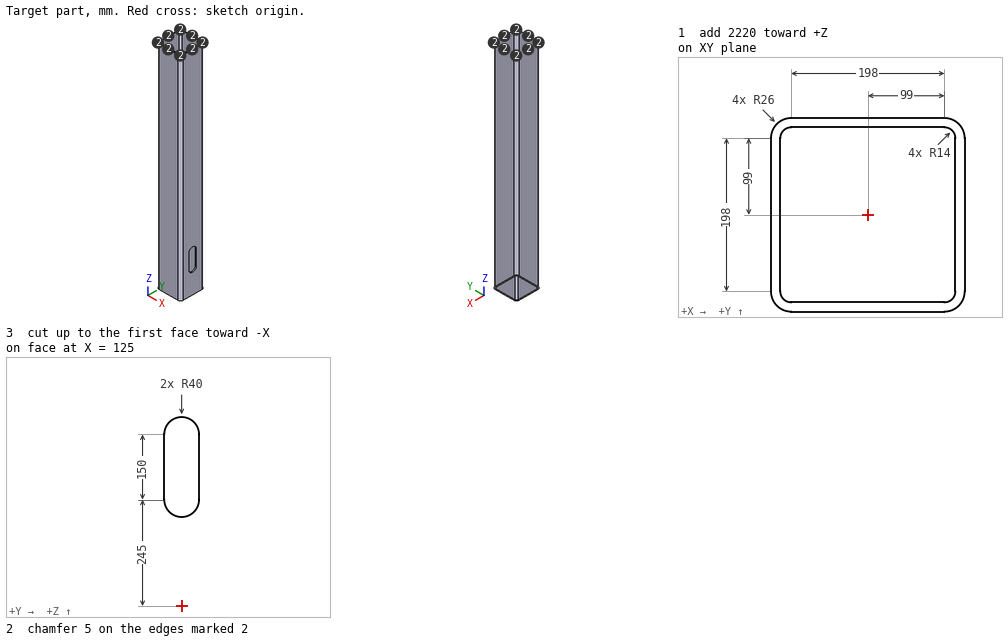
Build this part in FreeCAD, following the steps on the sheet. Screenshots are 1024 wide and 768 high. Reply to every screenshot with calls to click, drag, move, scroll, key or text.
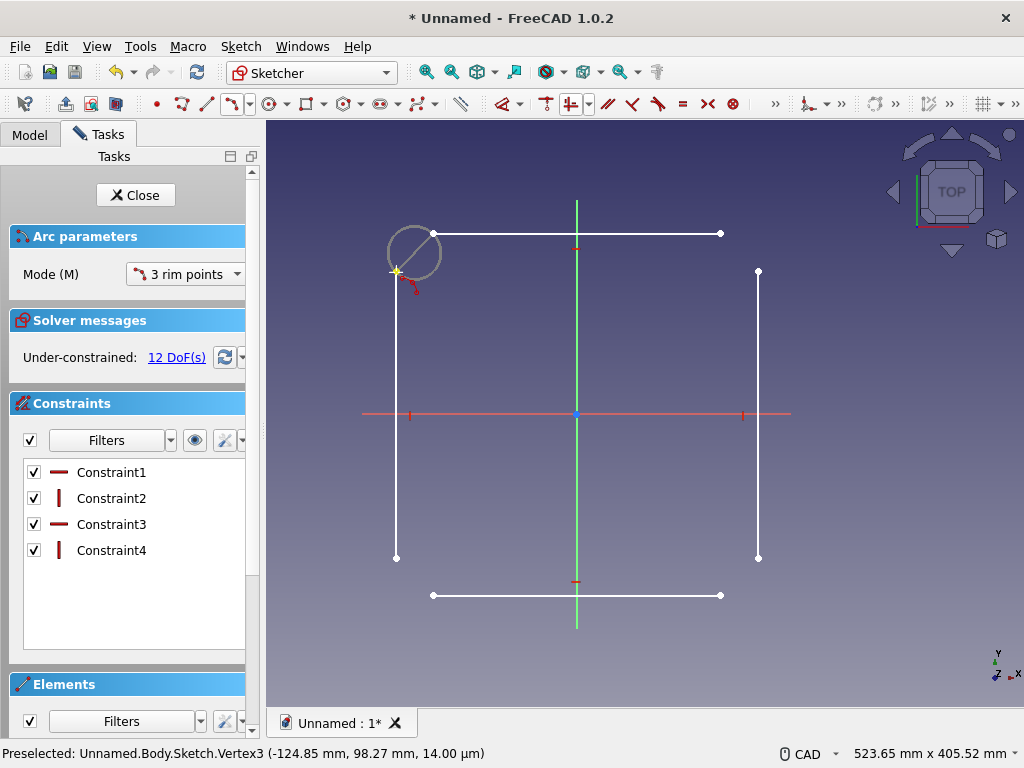
scroll(407, 244, up, 2)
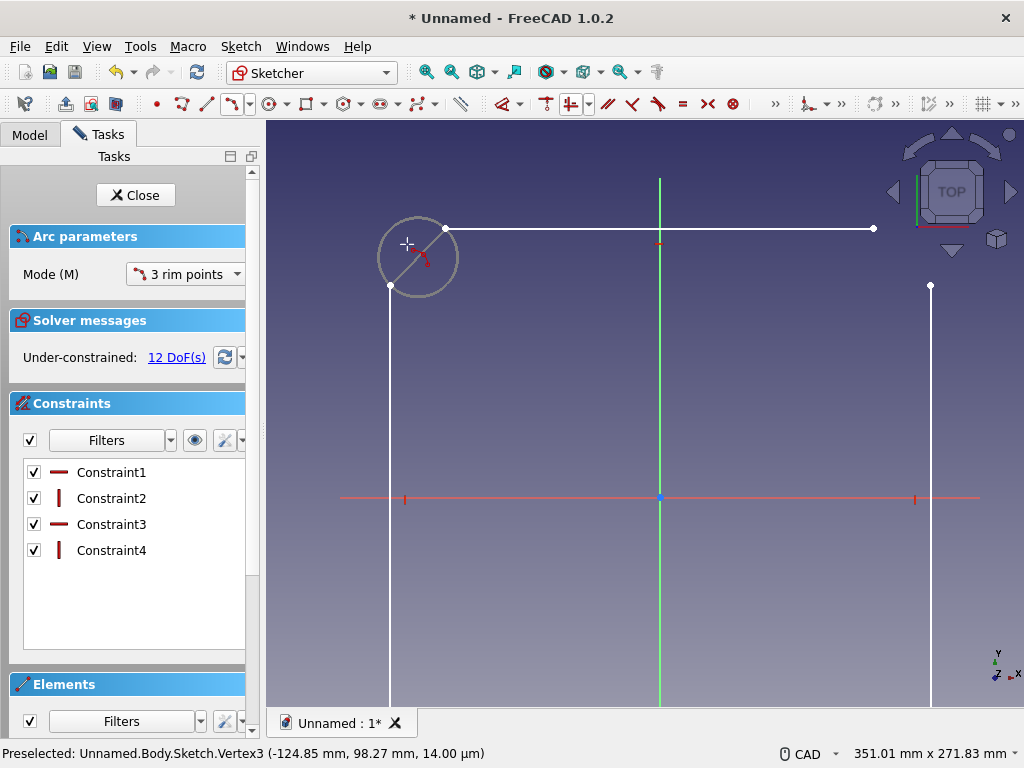
click(407, 244)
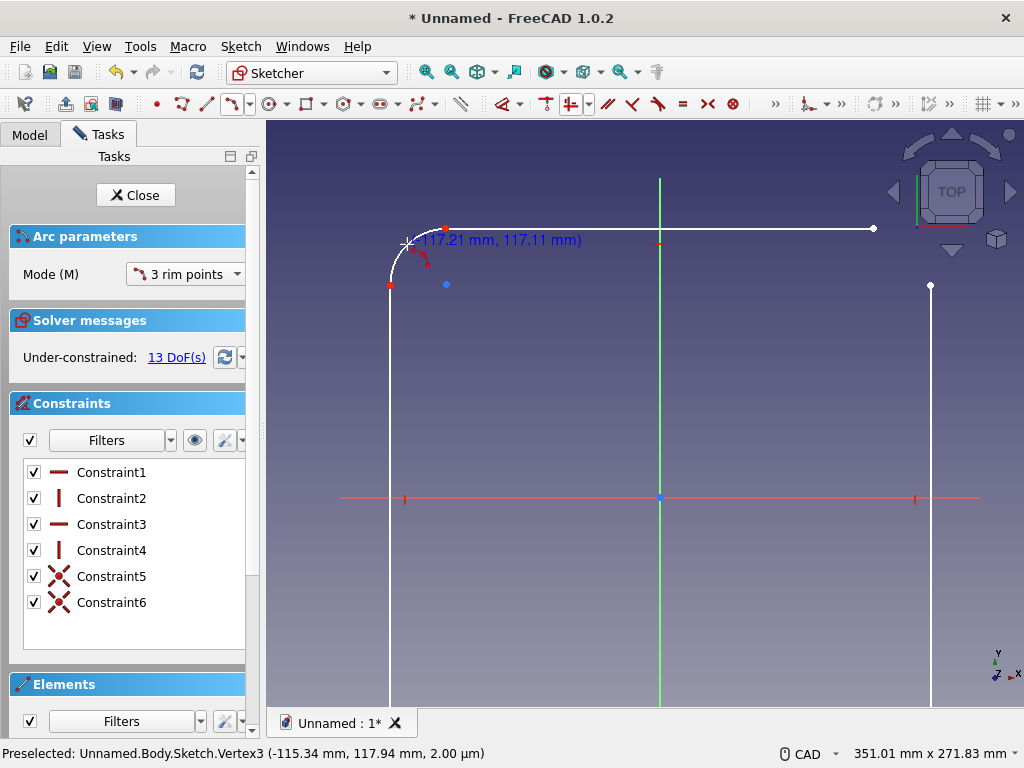
scroll(406, 242, down, 2)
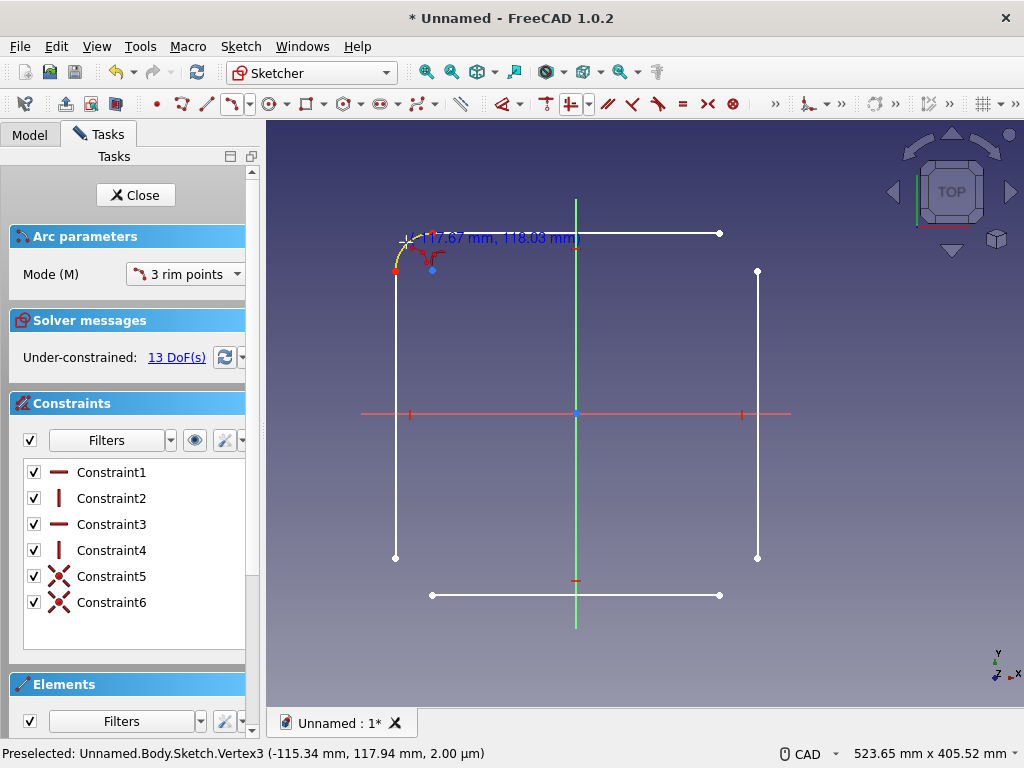
click(396, 558)
click(433, 595)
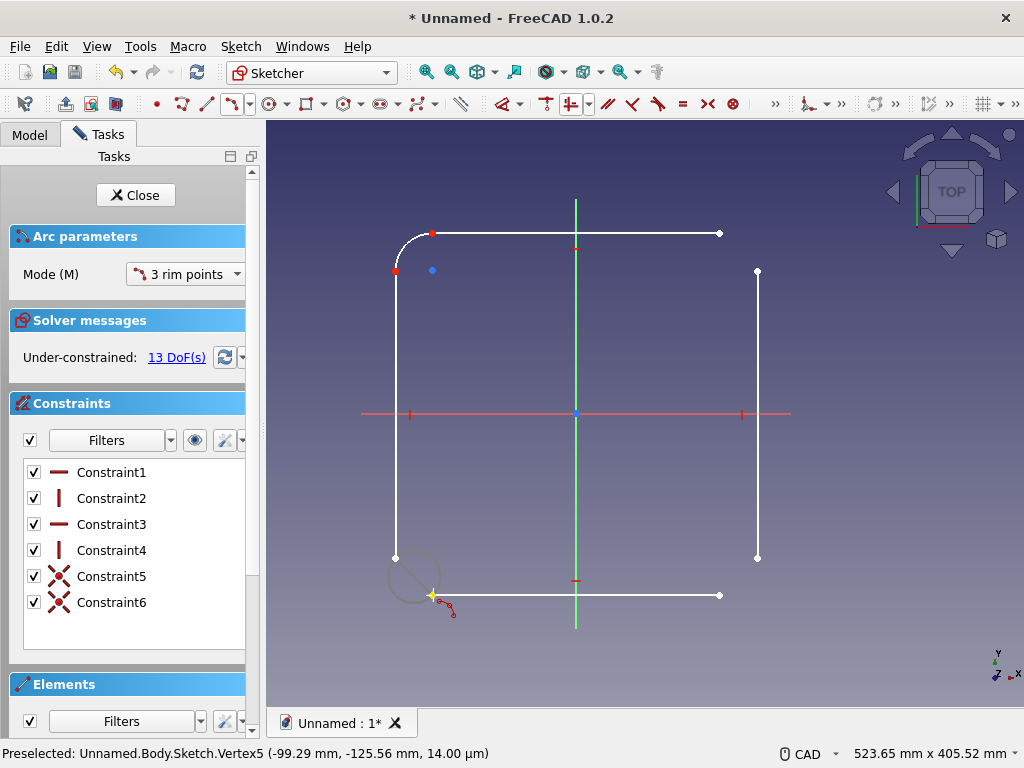
scroll(406, 584, up, 2)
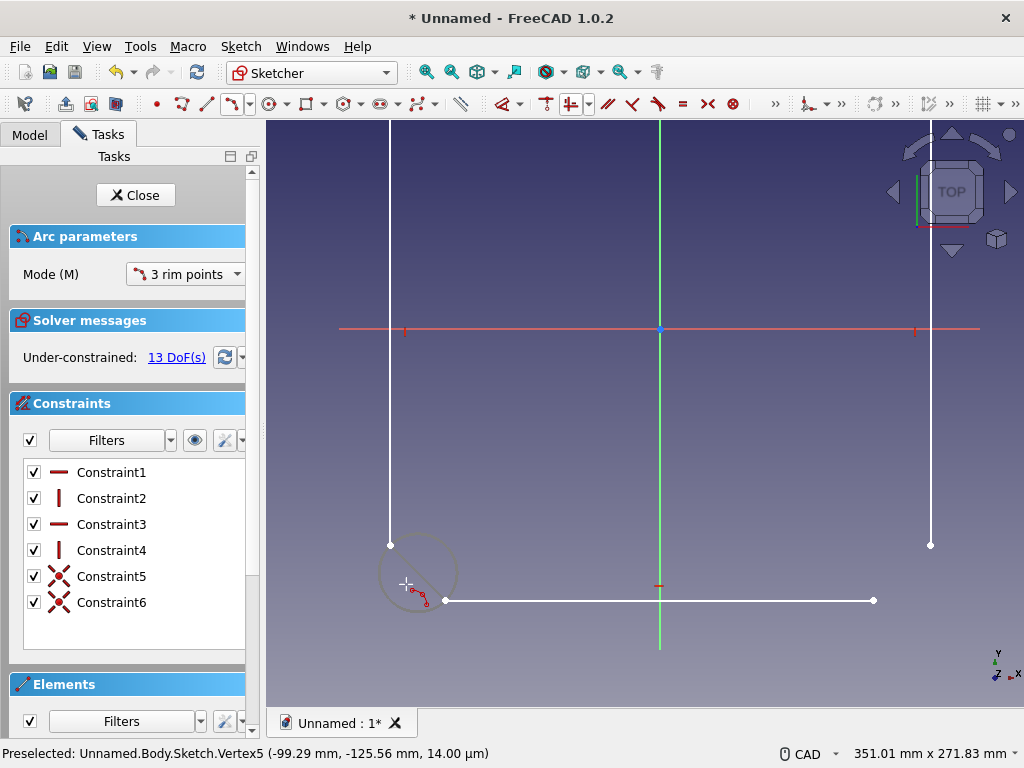
click(407, 583)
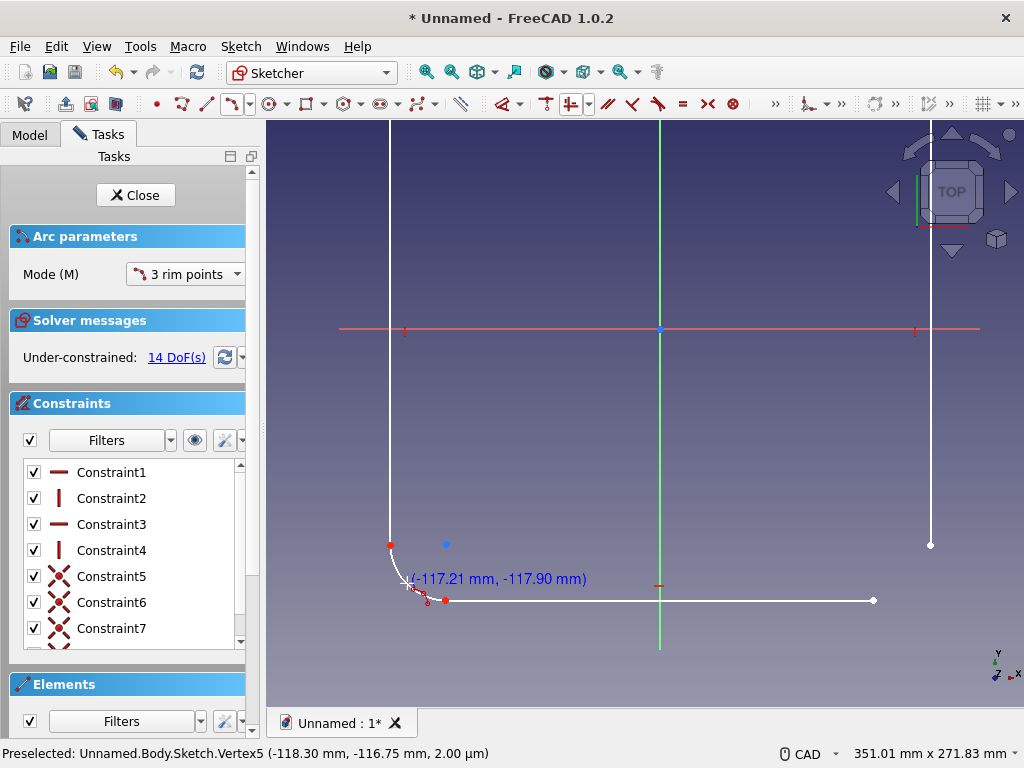
scroll(406, 585, down, 2)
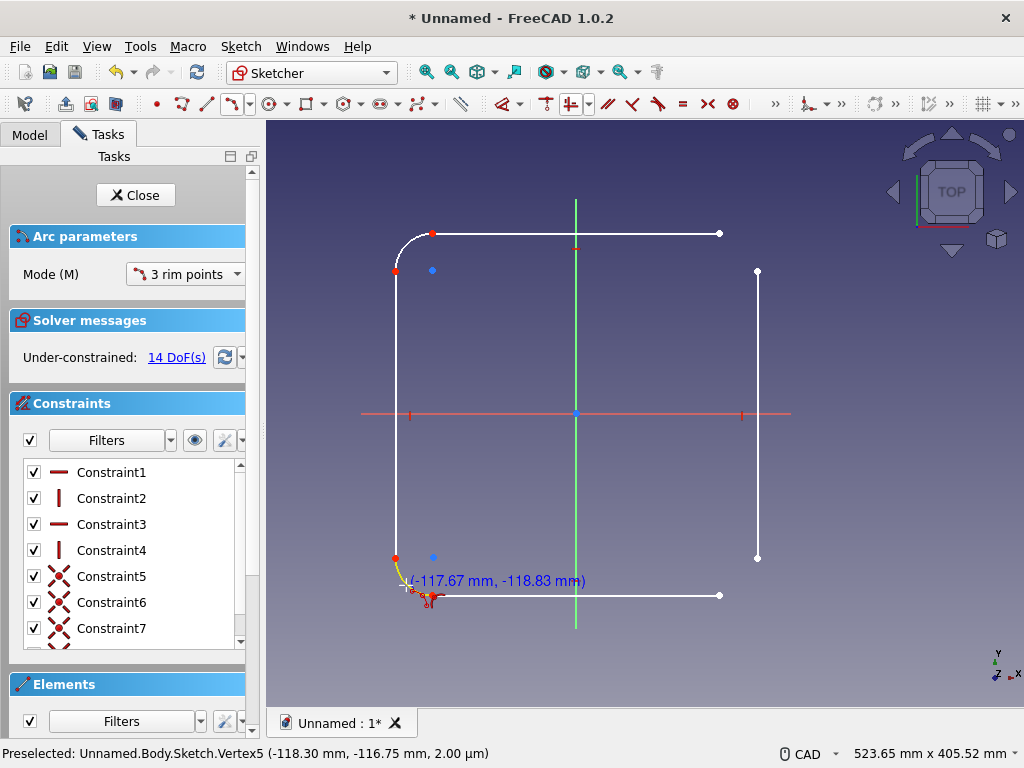
click(720, 596)
click(758, 559)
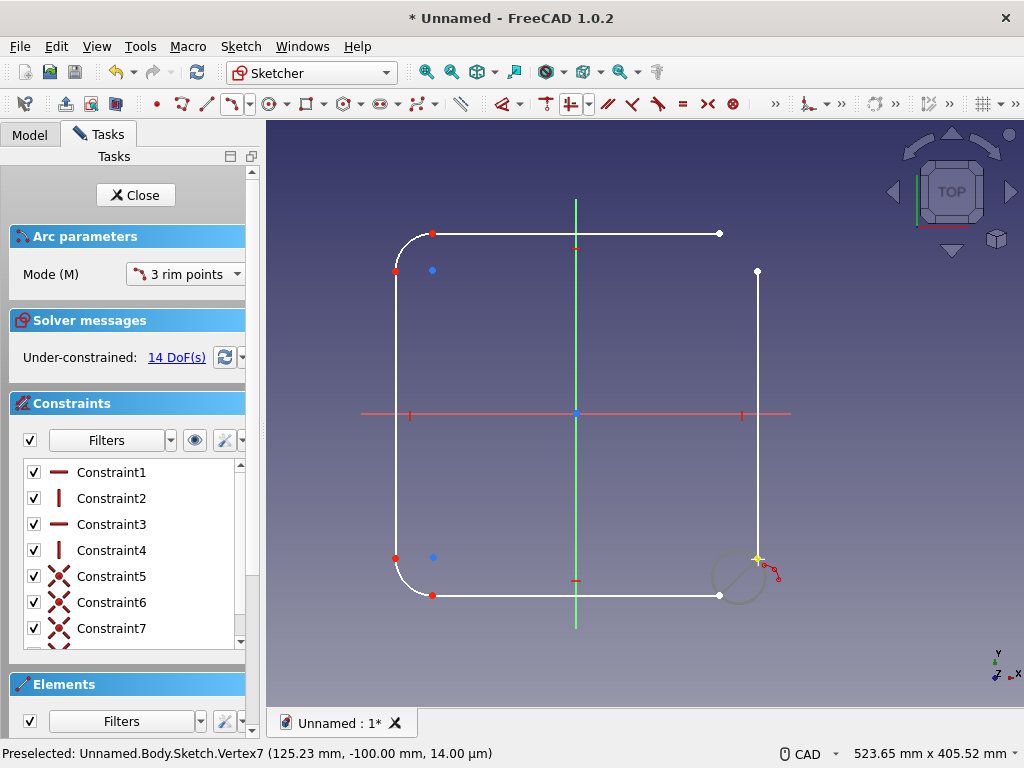
scroll(746, 584, up, 2)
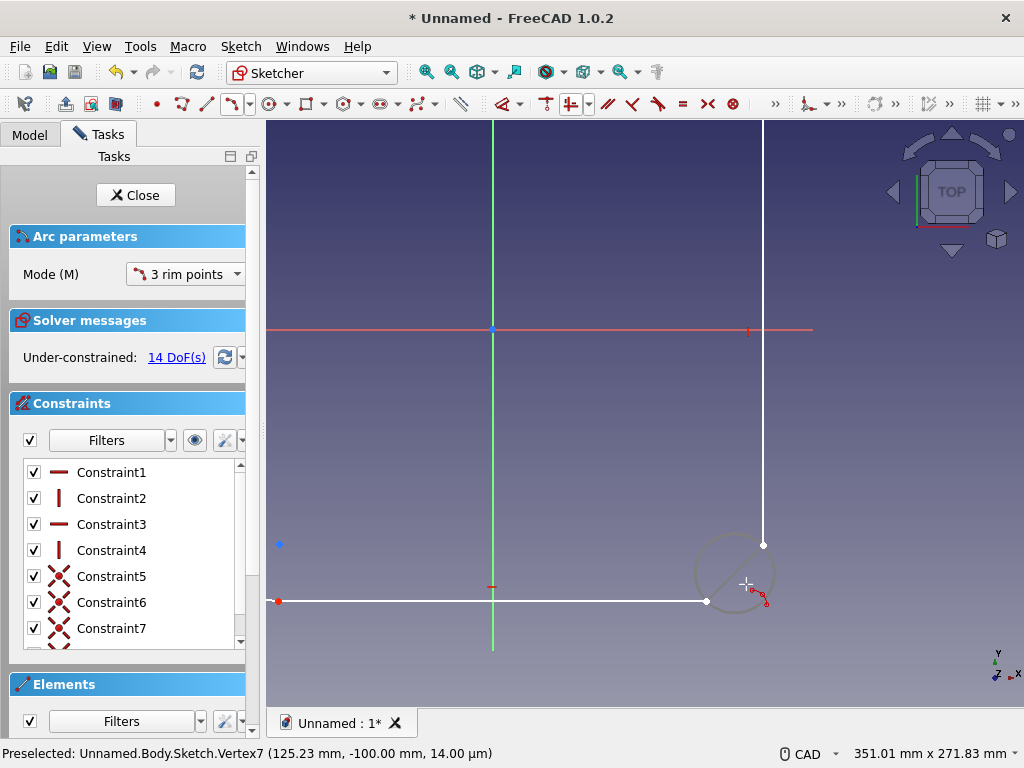
click(746, 583)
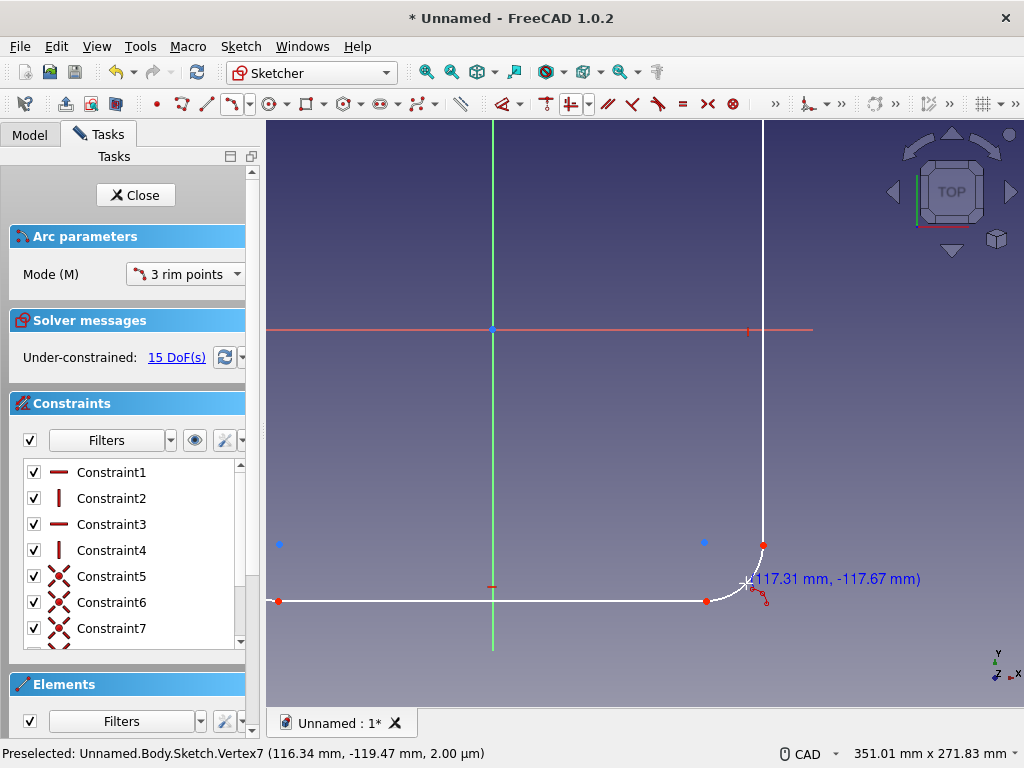
scroll(747, 584, down, 2)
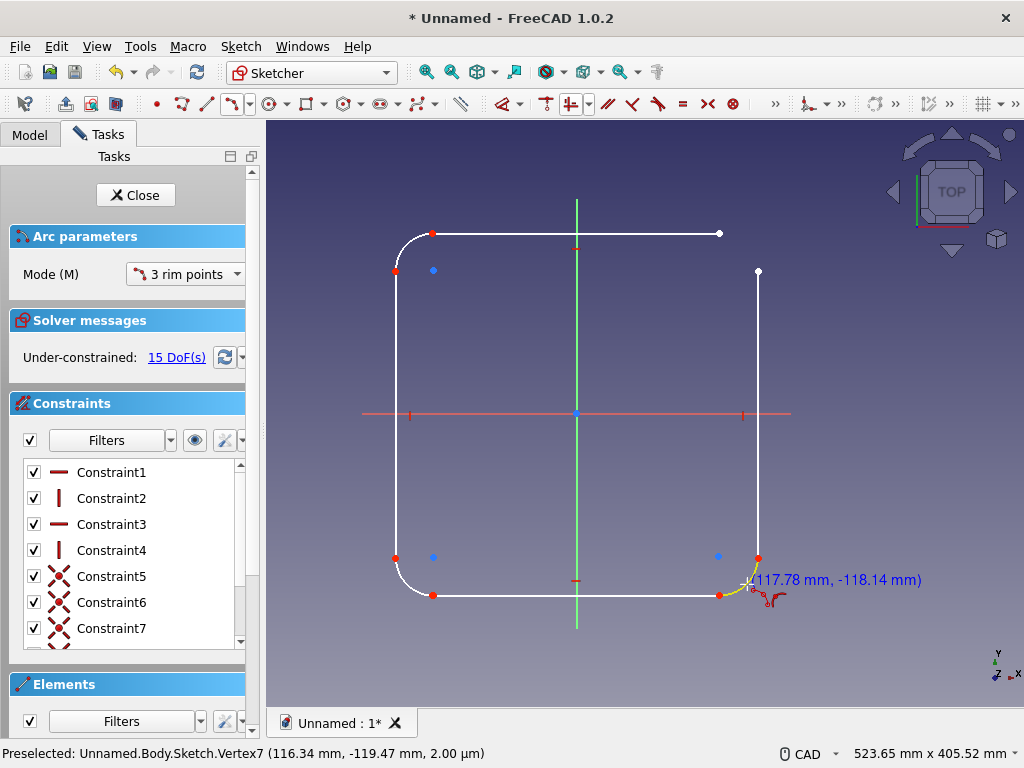
click(758, 272)
click(720, 234)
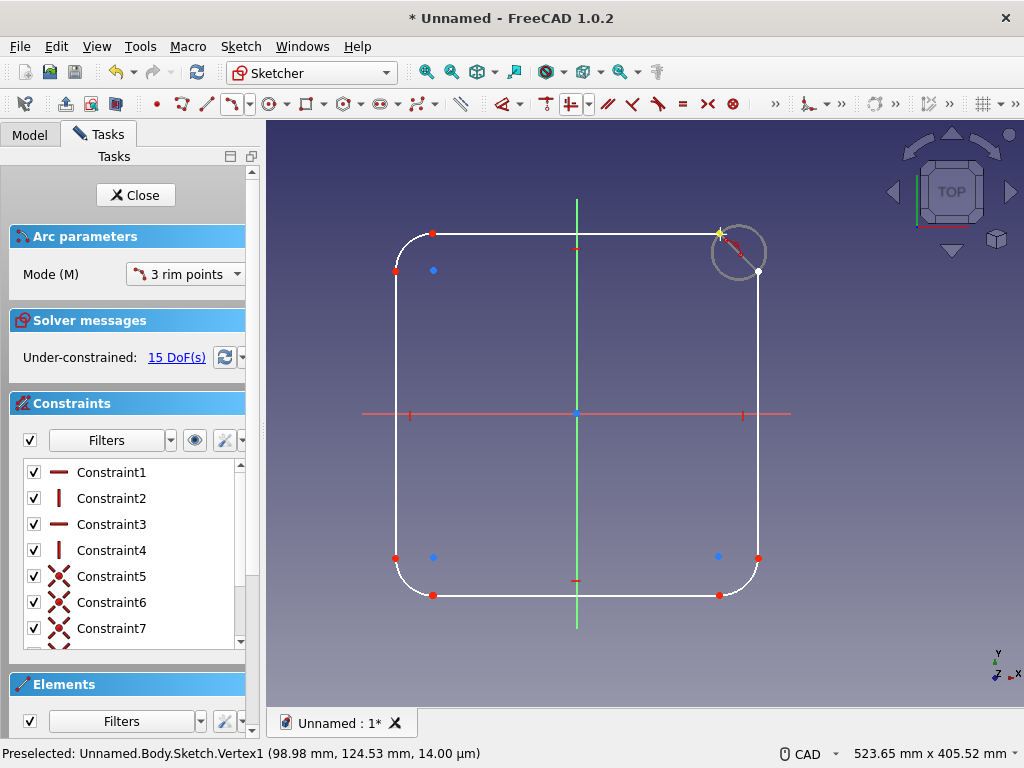
scroll(747, 244, up, 2)